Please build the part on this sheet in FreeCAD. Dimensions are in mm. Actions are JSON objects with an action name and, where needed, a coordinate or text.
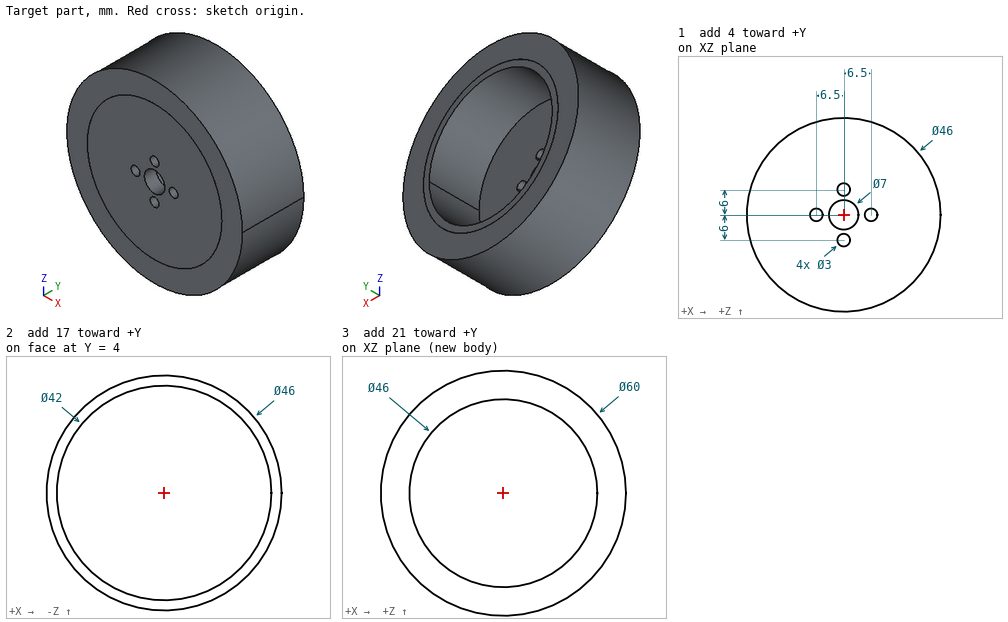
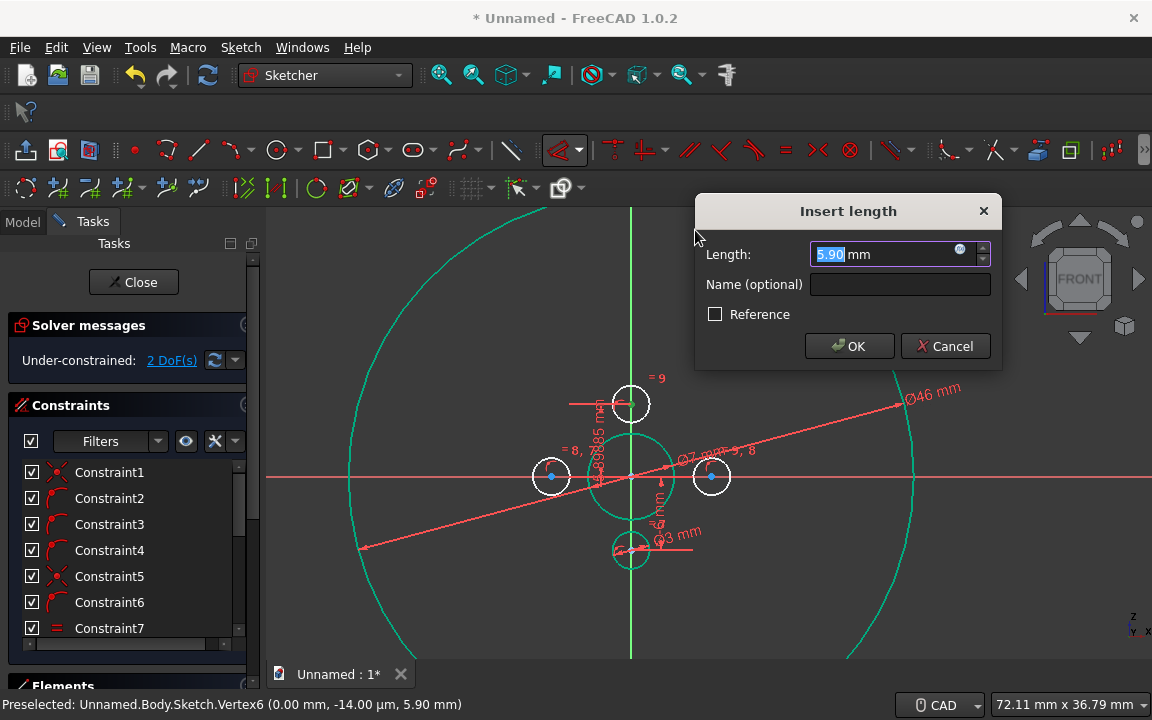
{"action": "type", "text": "6"}
{"action": "key", "text": "Return"}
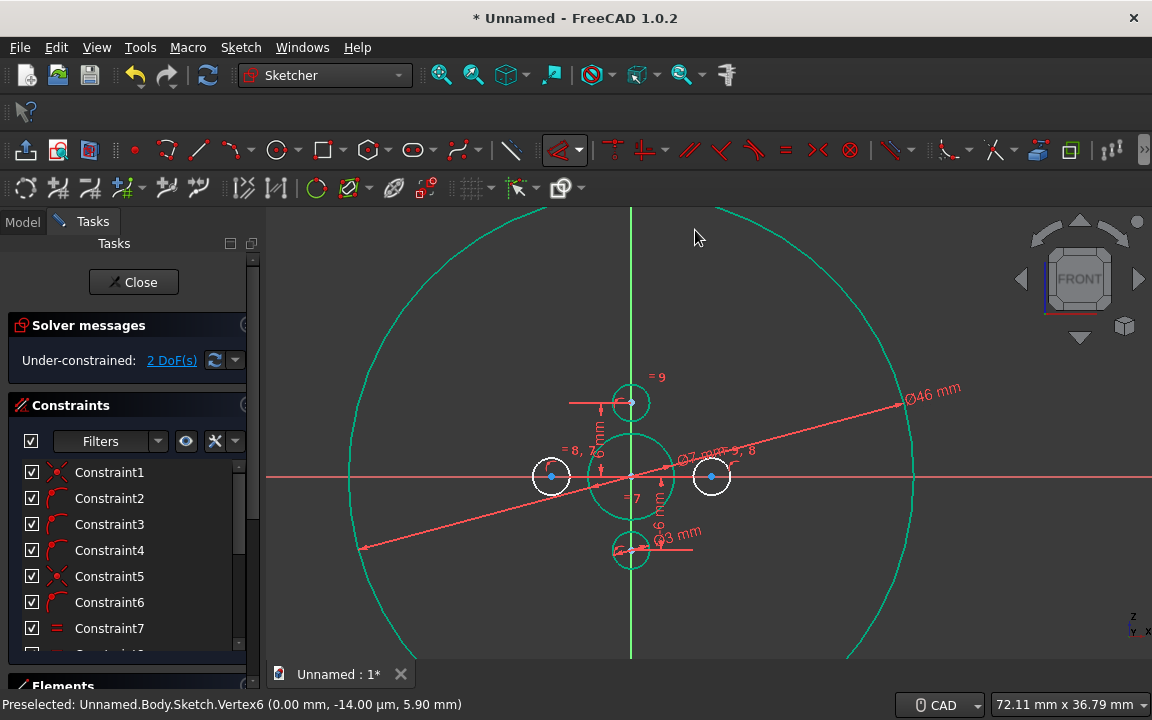
{"action": "left_click", "coordinate": [551, 477]}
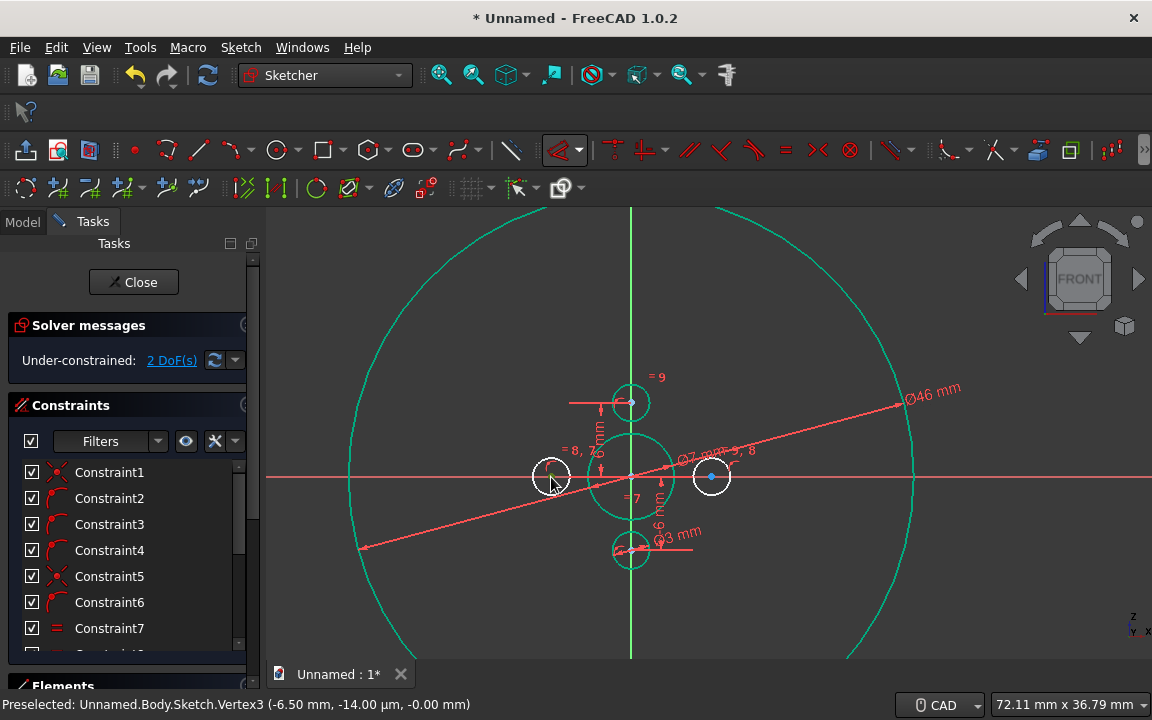
{"action": "left_click", "coordinate": [582, 150]}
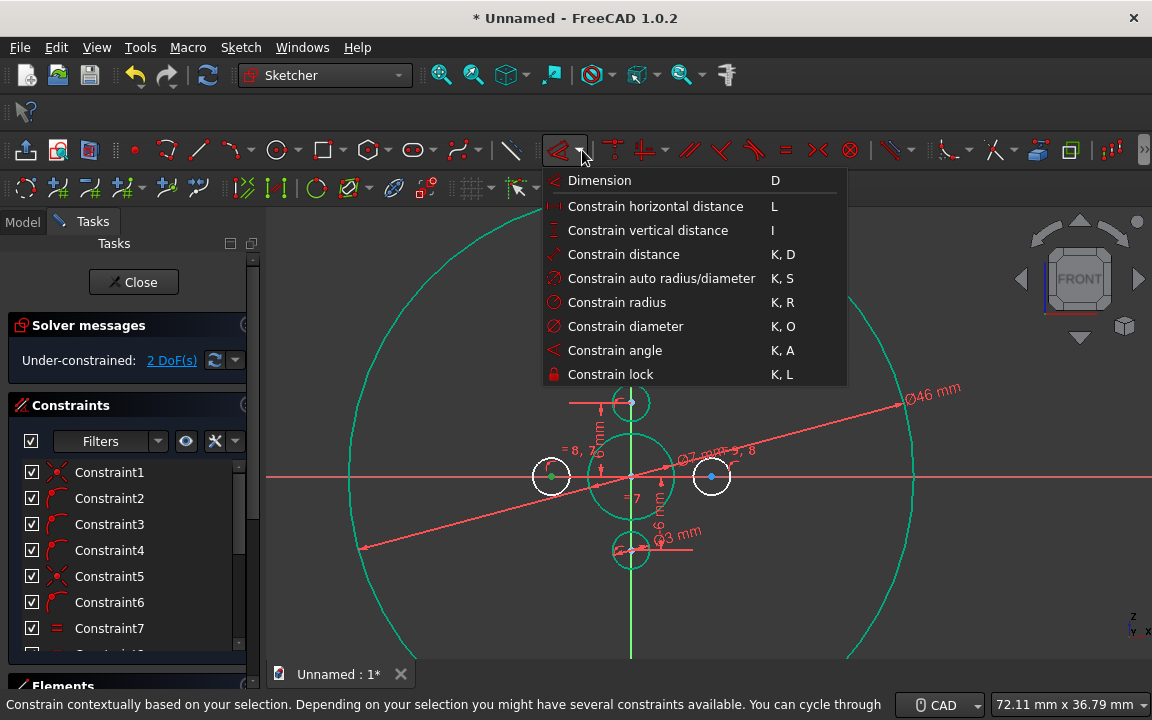
{"action": "left_click", "coordinate": [695, 206]}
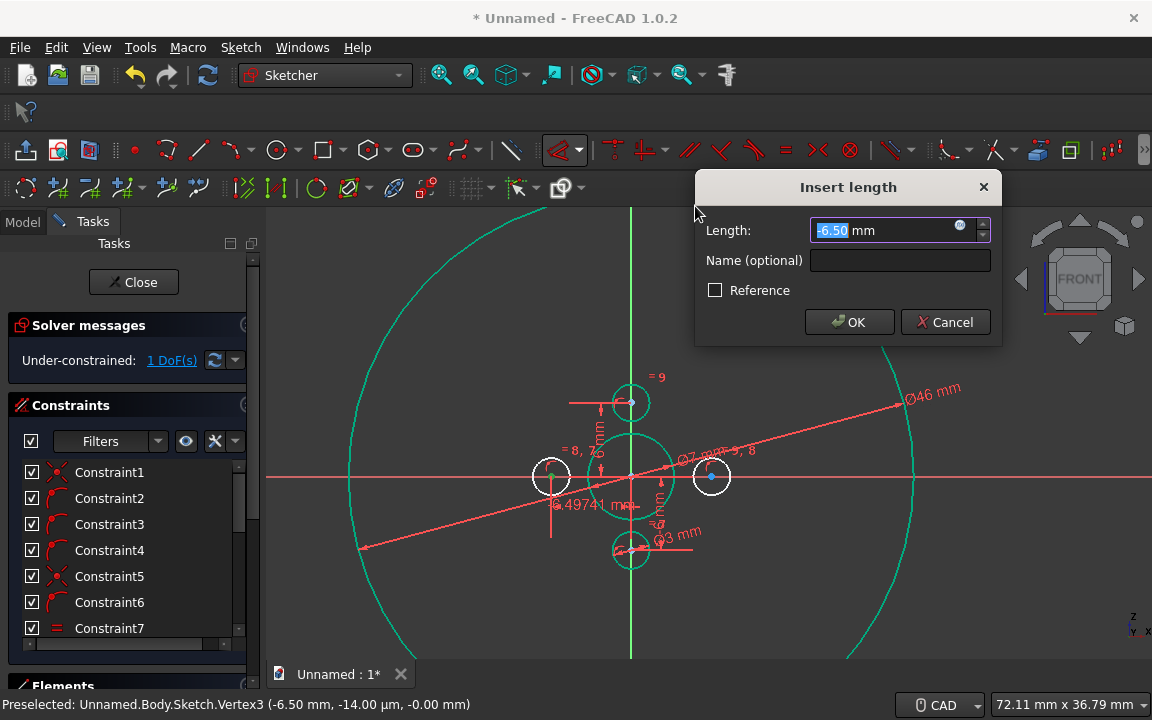
{"action": "type", "text": "-6.5"}
{"action": "key", "text": "Return"}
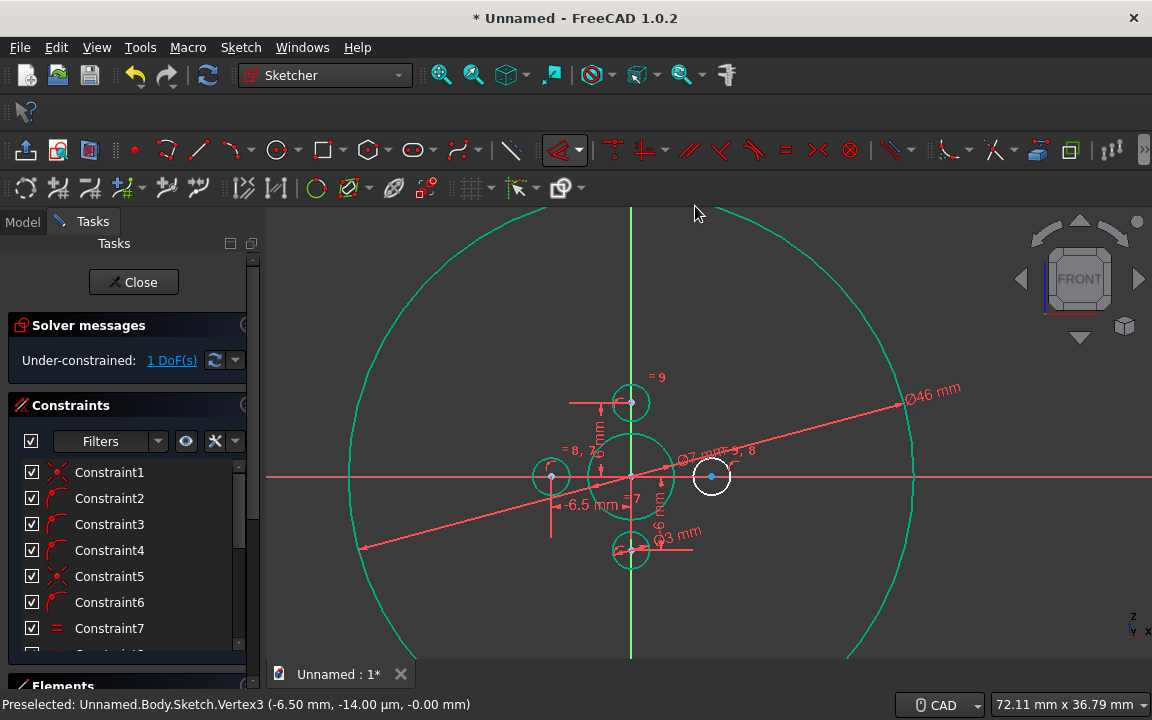
{"action": "left_click", "coordinate": [712, 477]}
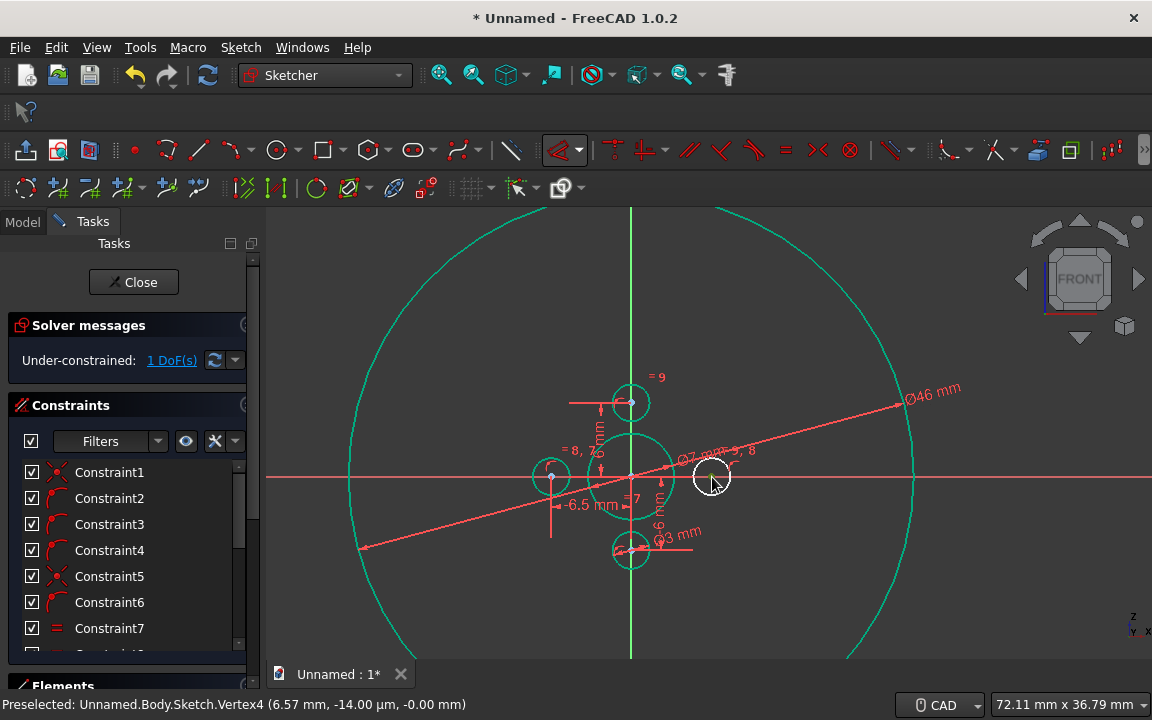
{"action": "key", "text": "l"}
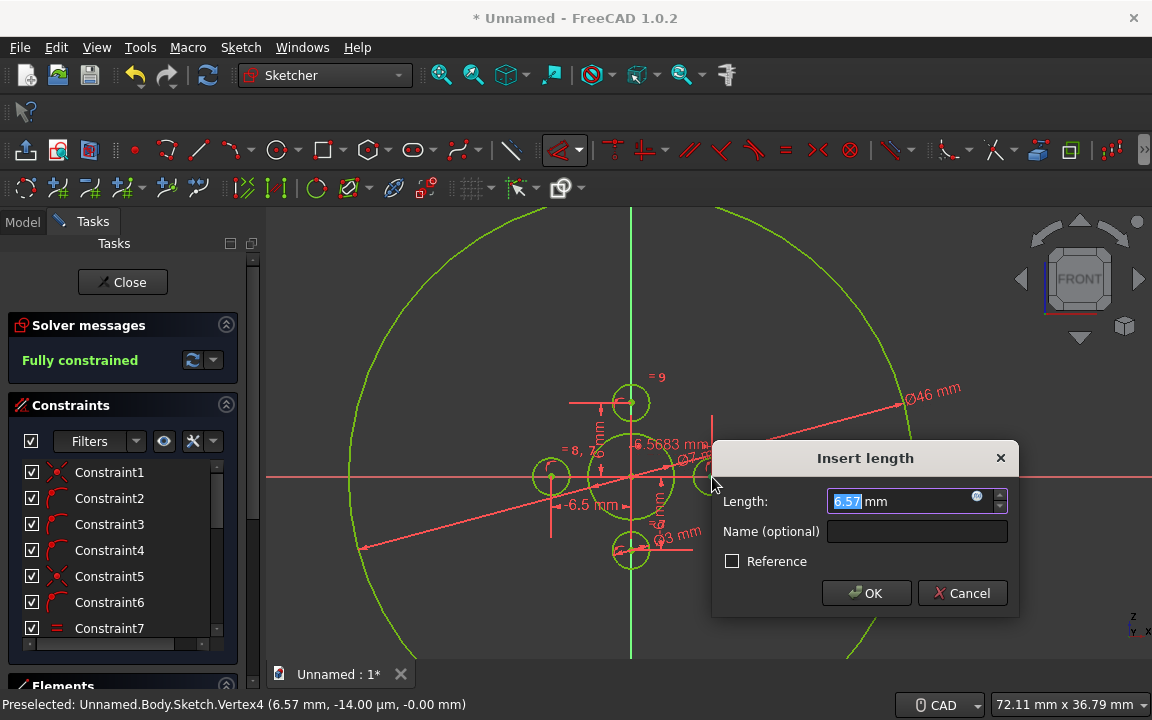
{"action": "type", "text": "6.5"}
{"action": "key", "text": "Return"}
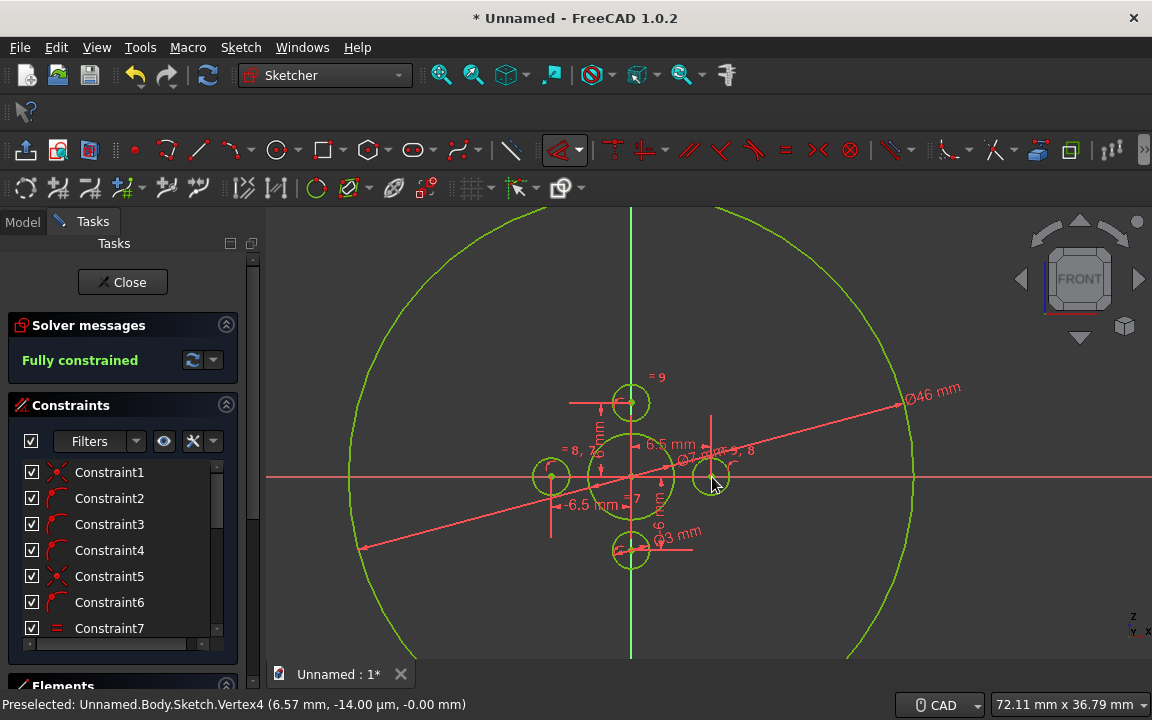
{"action": "left_click", "coordinate": [123, 282]}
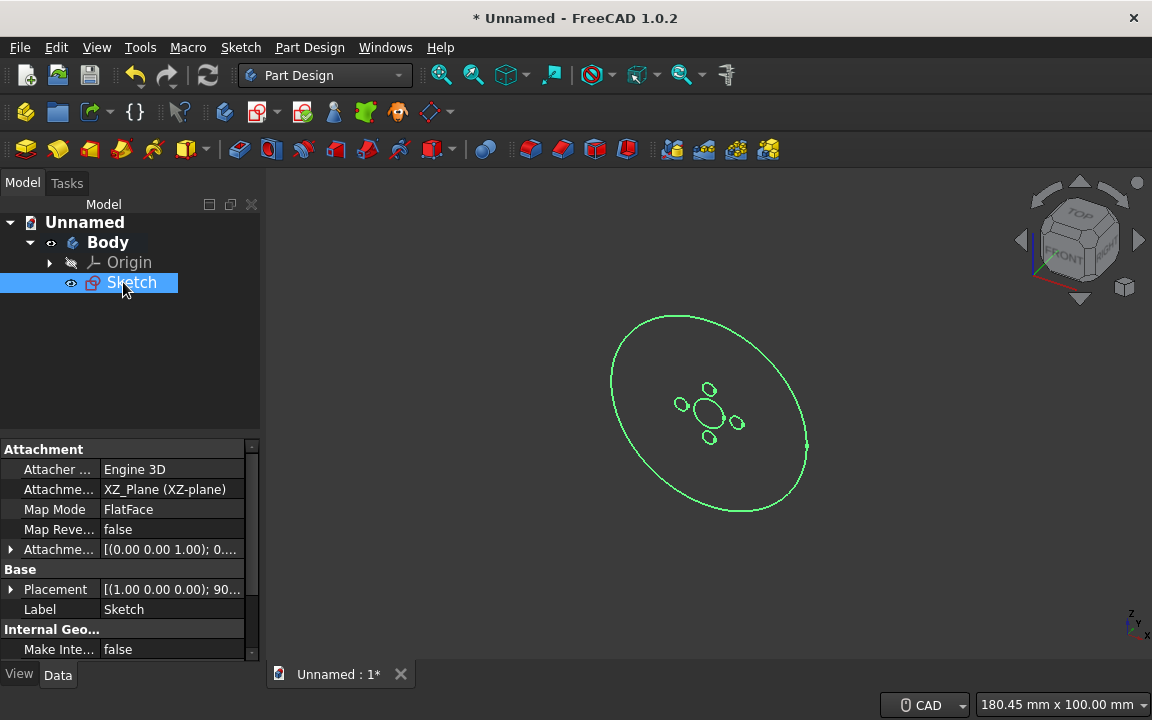
{"action": "left_click", "coordinate": [26, 150]}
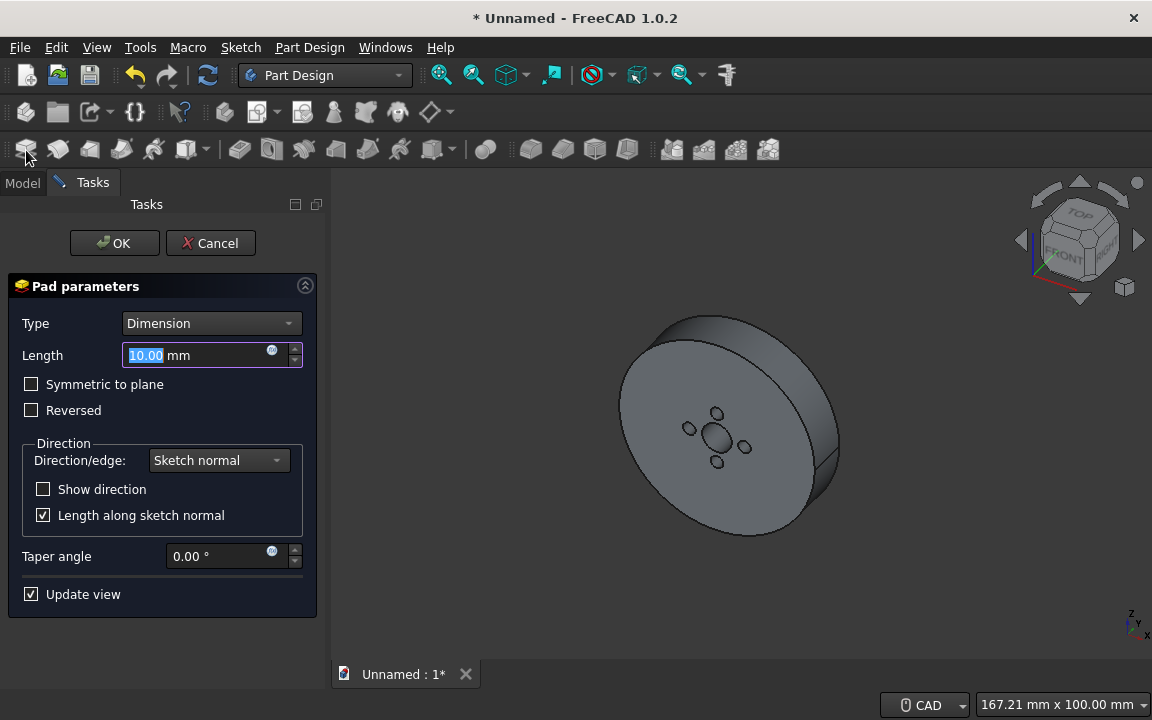
{"action": "type", "text": "4"}
{"action": "key", "text": "Tab"}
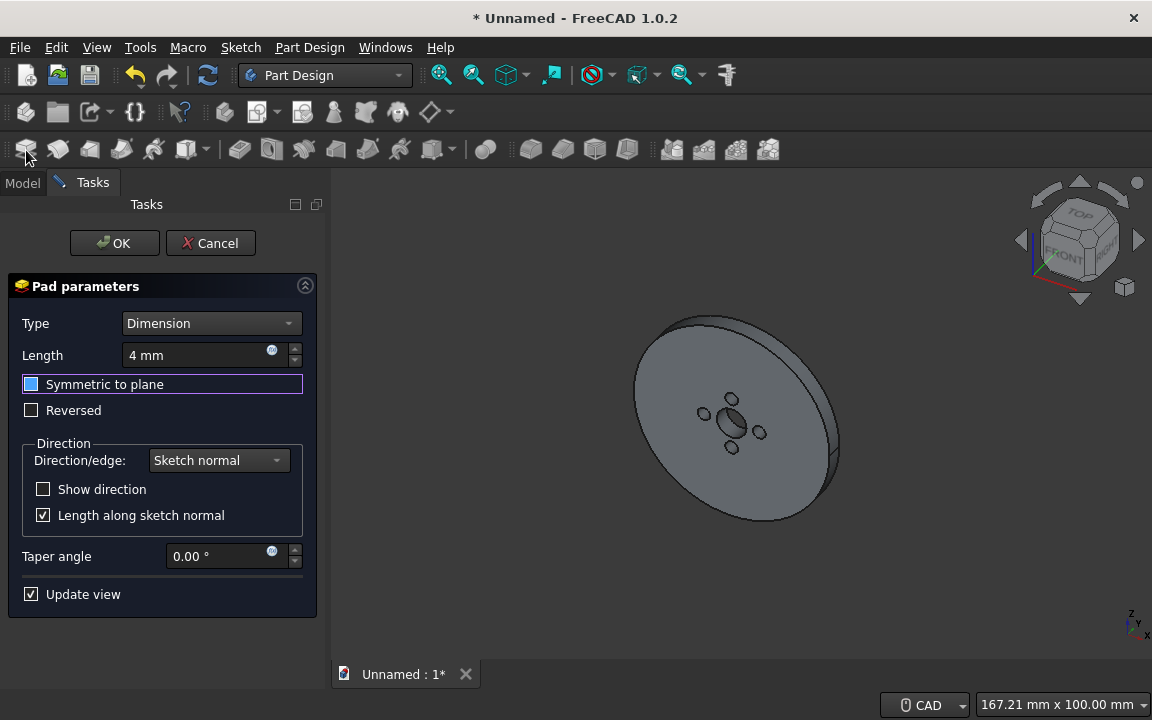
{"action": "left_click", "coordinate": [30, 410]}